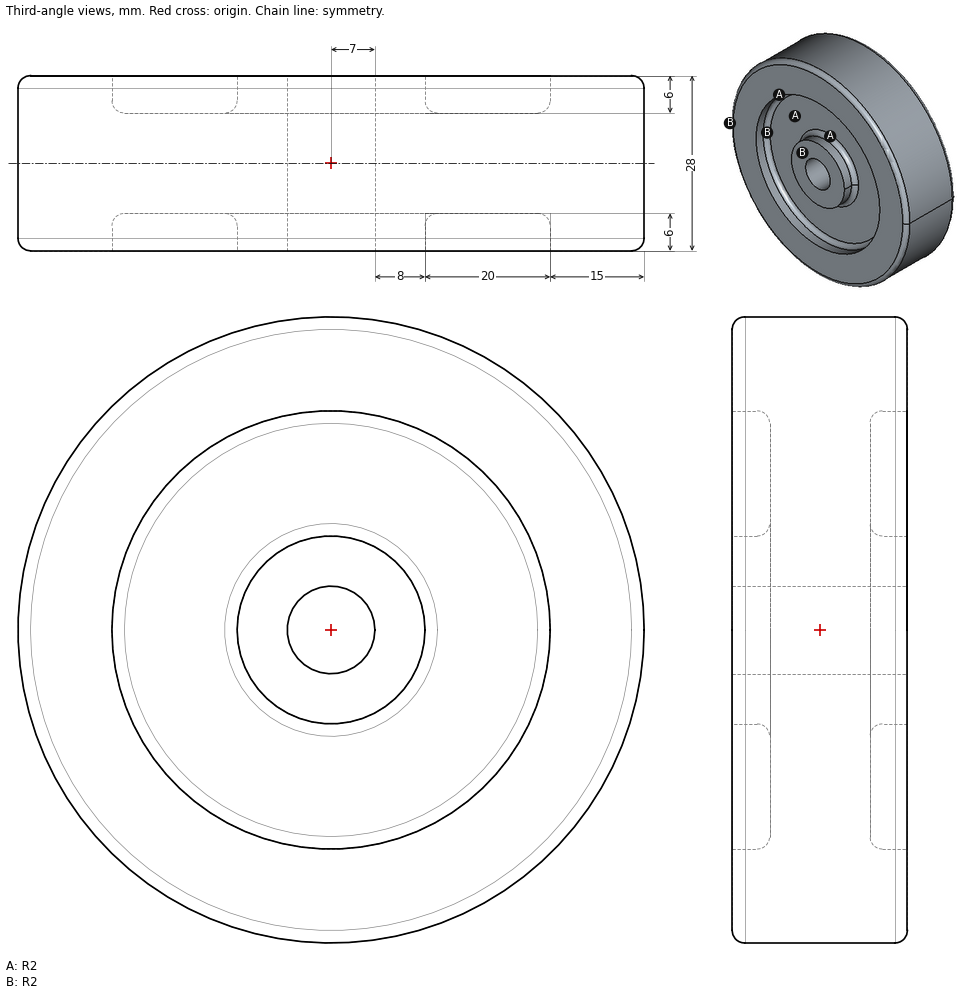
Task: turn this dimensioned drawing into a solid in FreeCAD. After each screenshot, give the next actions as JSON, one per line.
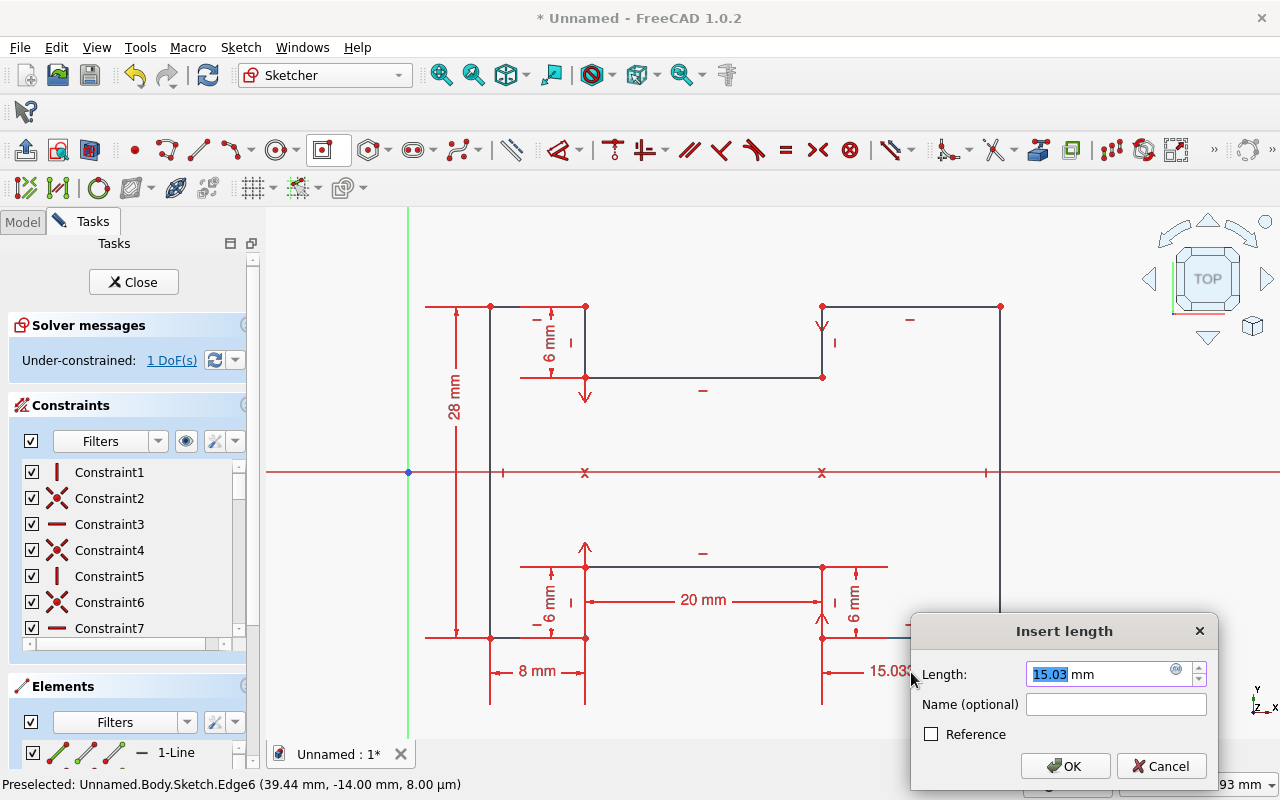
{"action": "type", "text": "15"}
{"action": "key", "text": "Return"}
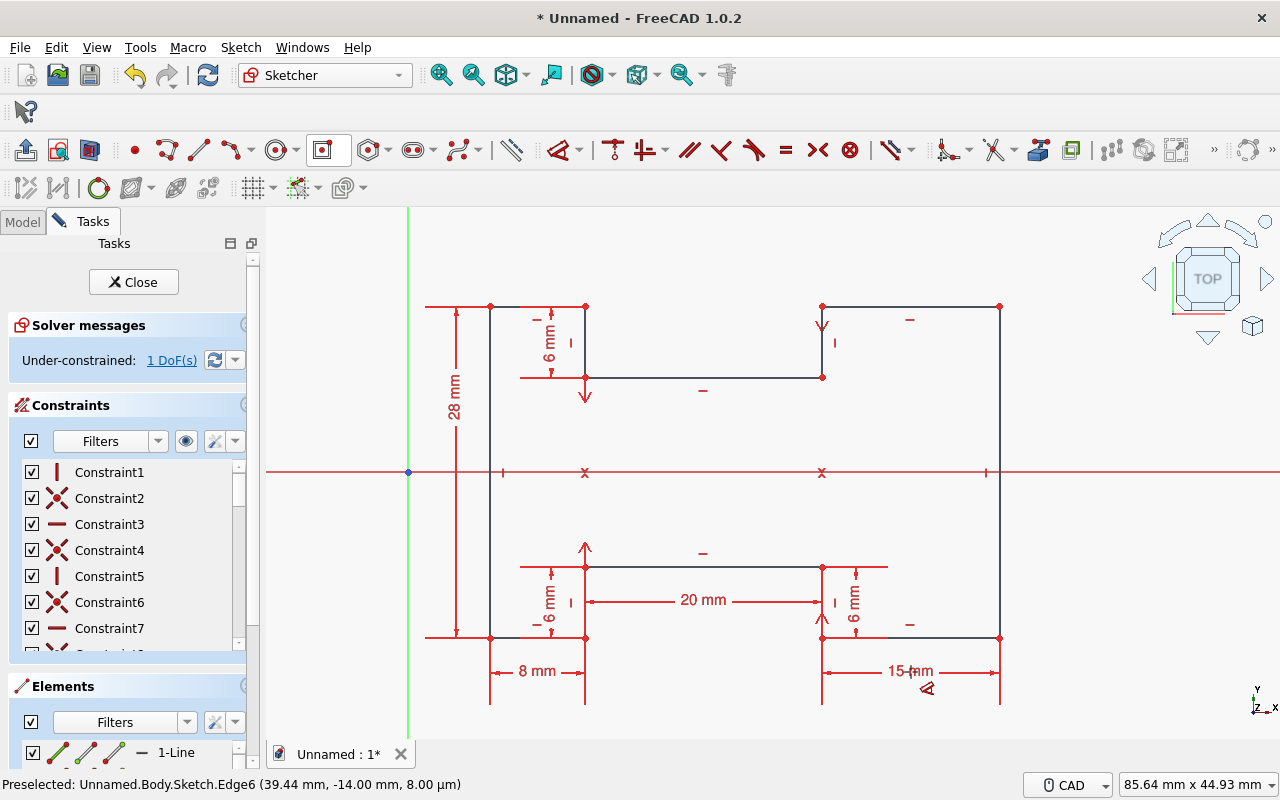
{"action": "left_click", "coordinate": [490, 307]}
{"action": "left_click", "coordinate": [449, 273]}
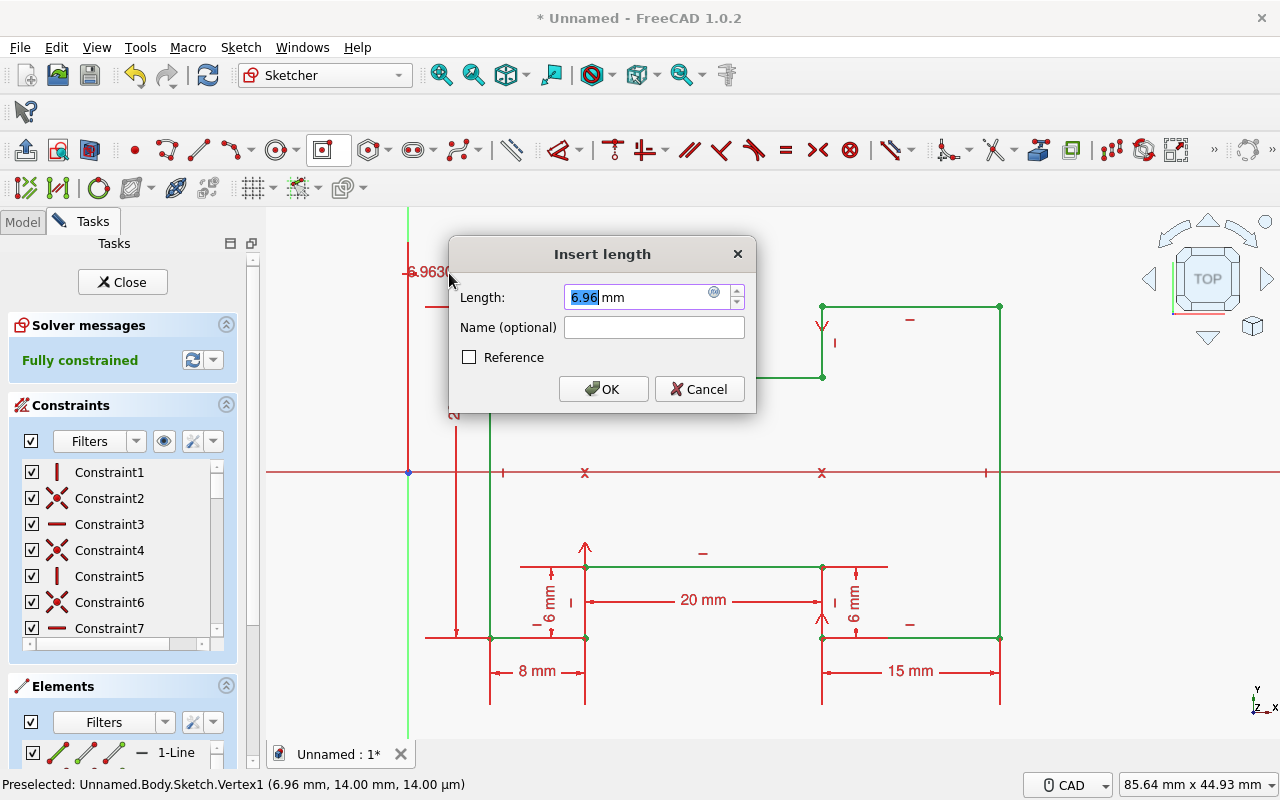
{"action": "type", "text": "7"}
{"action": "key", "text": "Return"}
{"action": "key", "text": "Escape"}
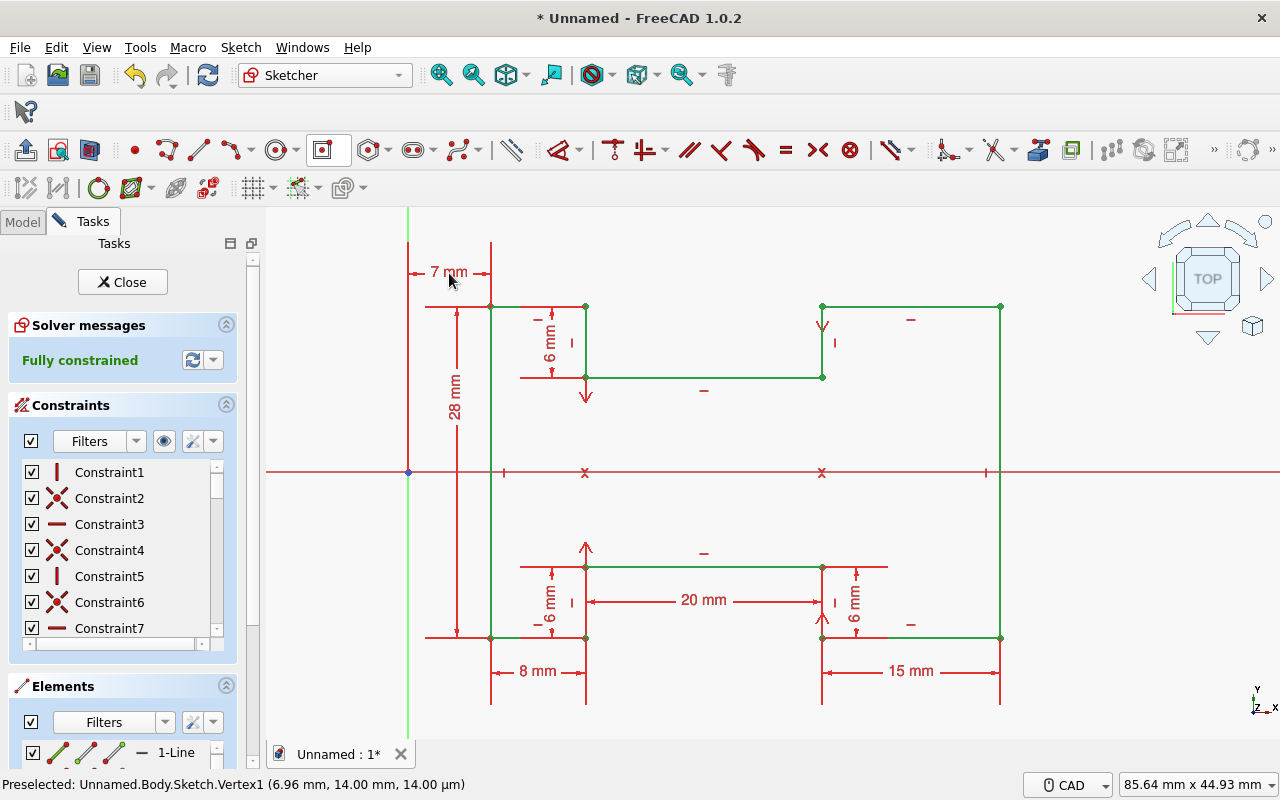
{"action": "left_click", "coordinate": [123, 282]}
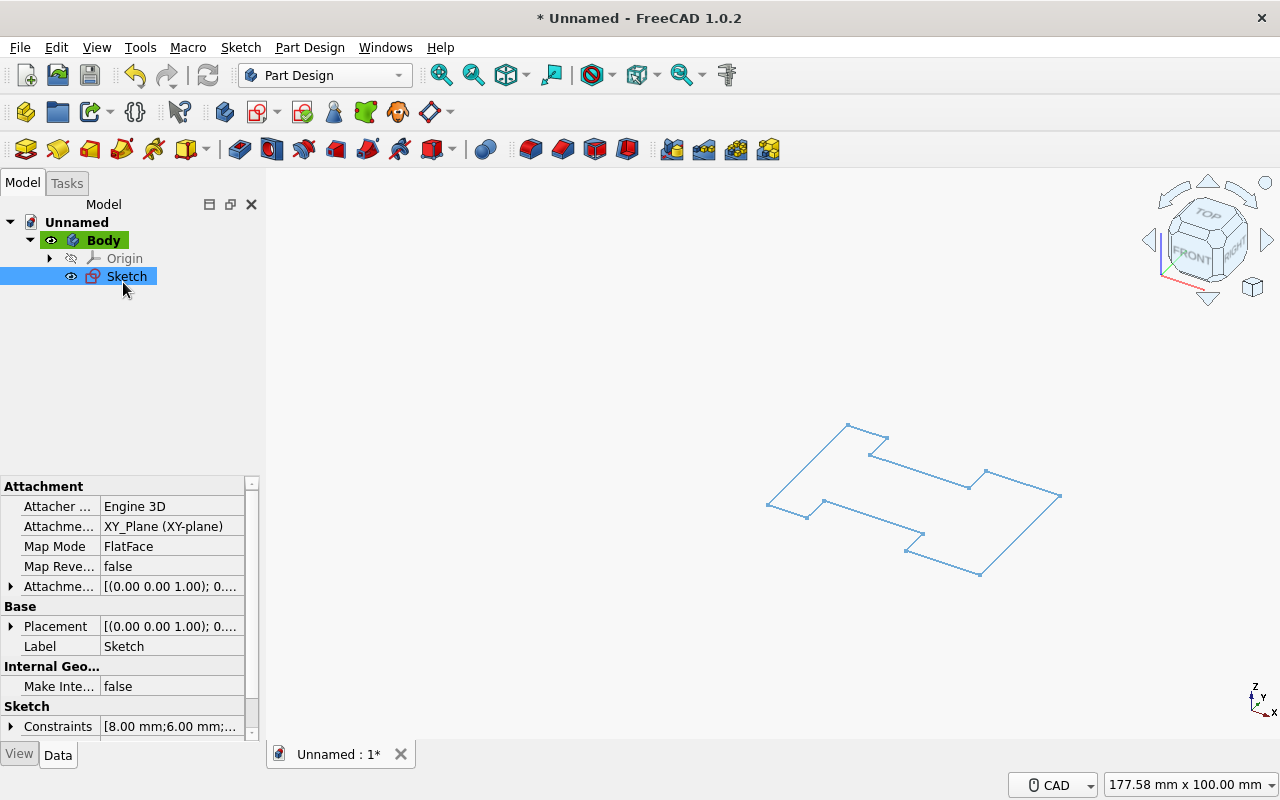
{"action": "left_click", "coordinate": [58, 150]}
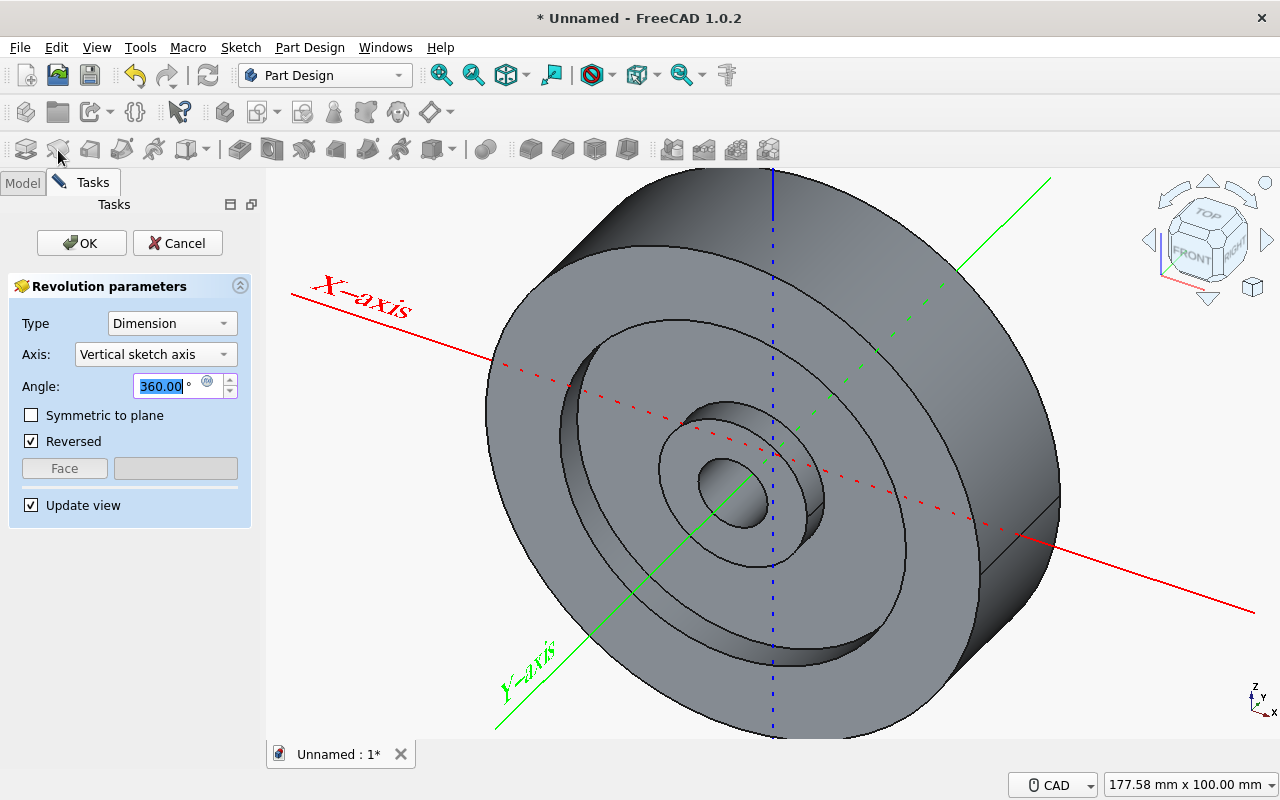
{"action": "left_click", "coordinate": [82, 243]}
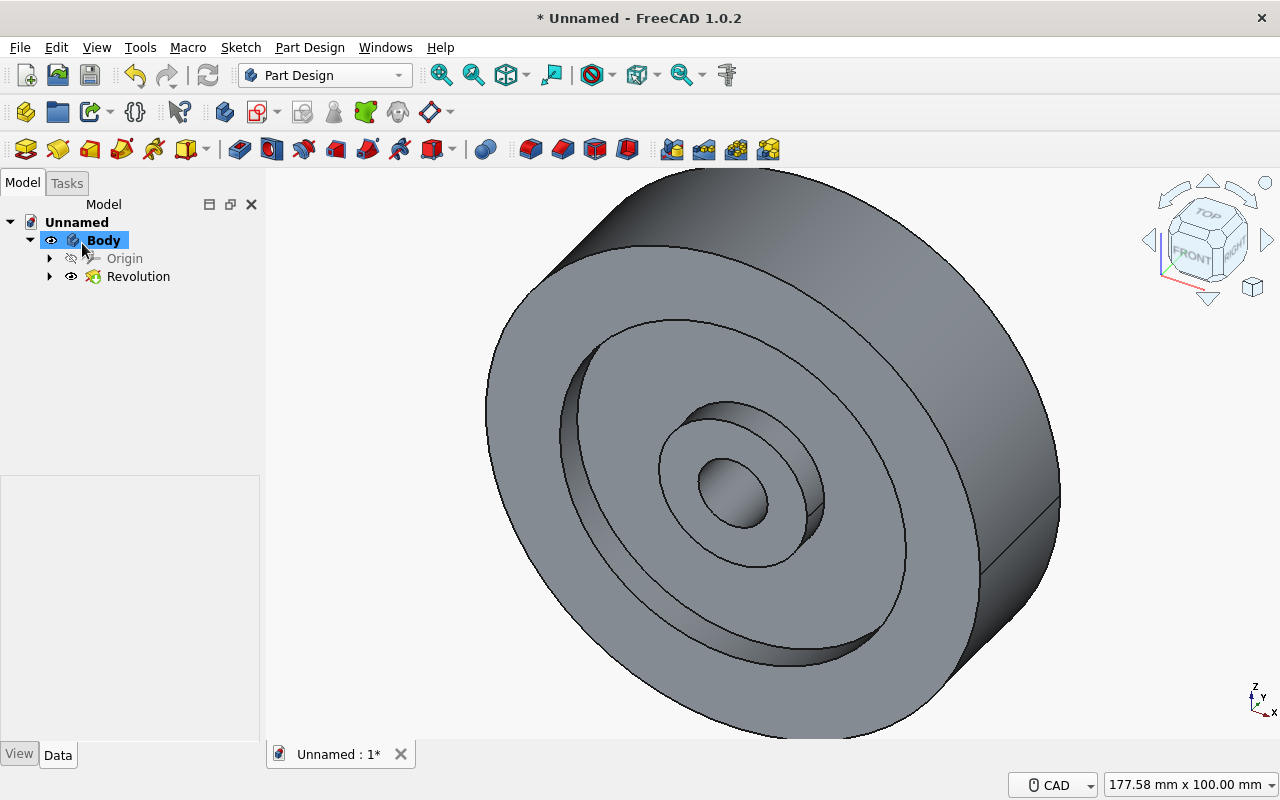
{"action": "left_click", "coordinate": [442, 76]}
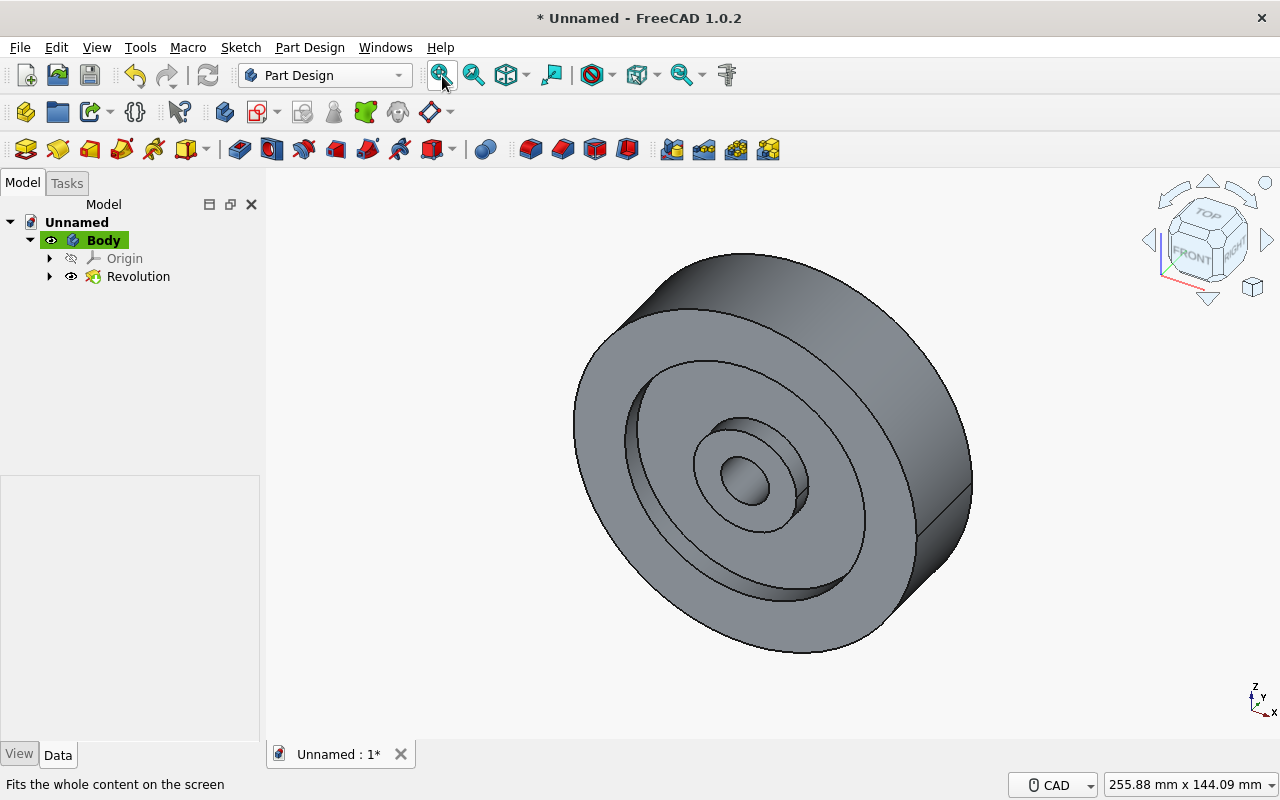
{"action": "key", "text": "0"}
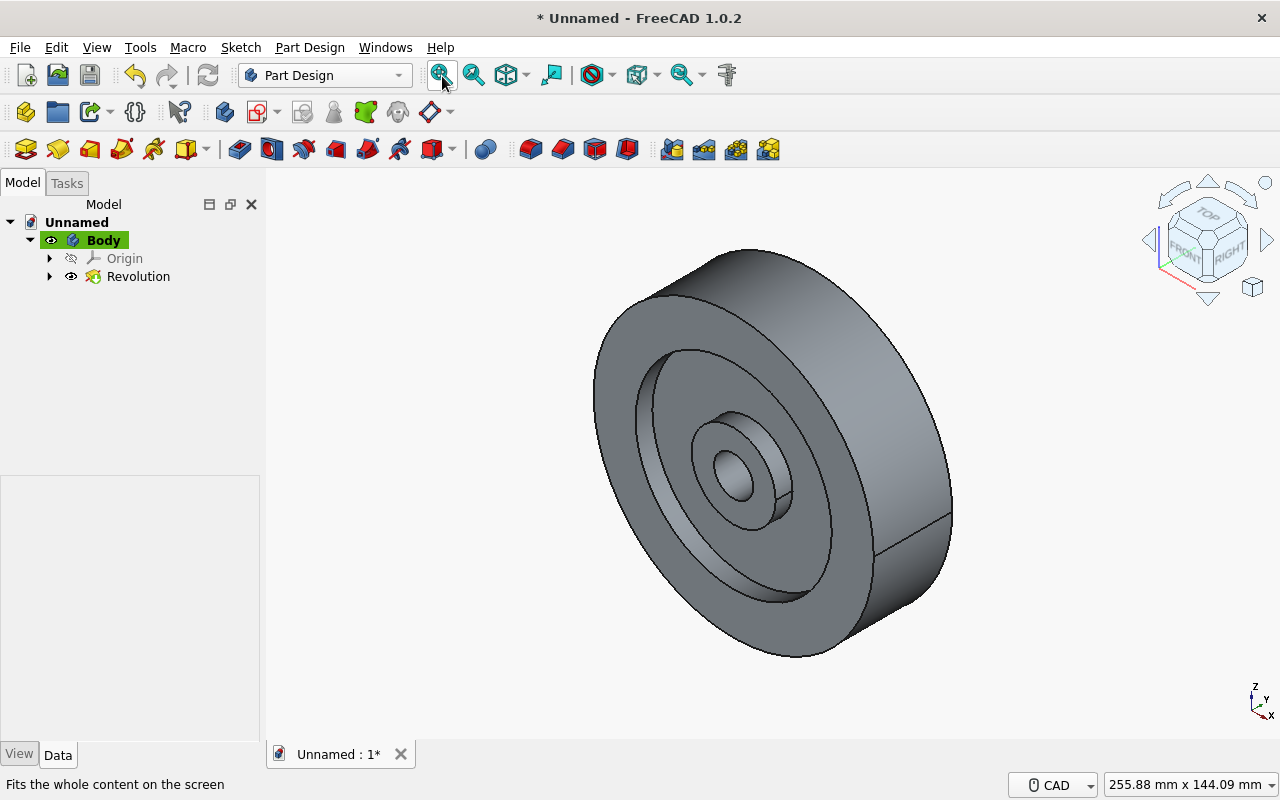
{"action": "key", "text": "2"}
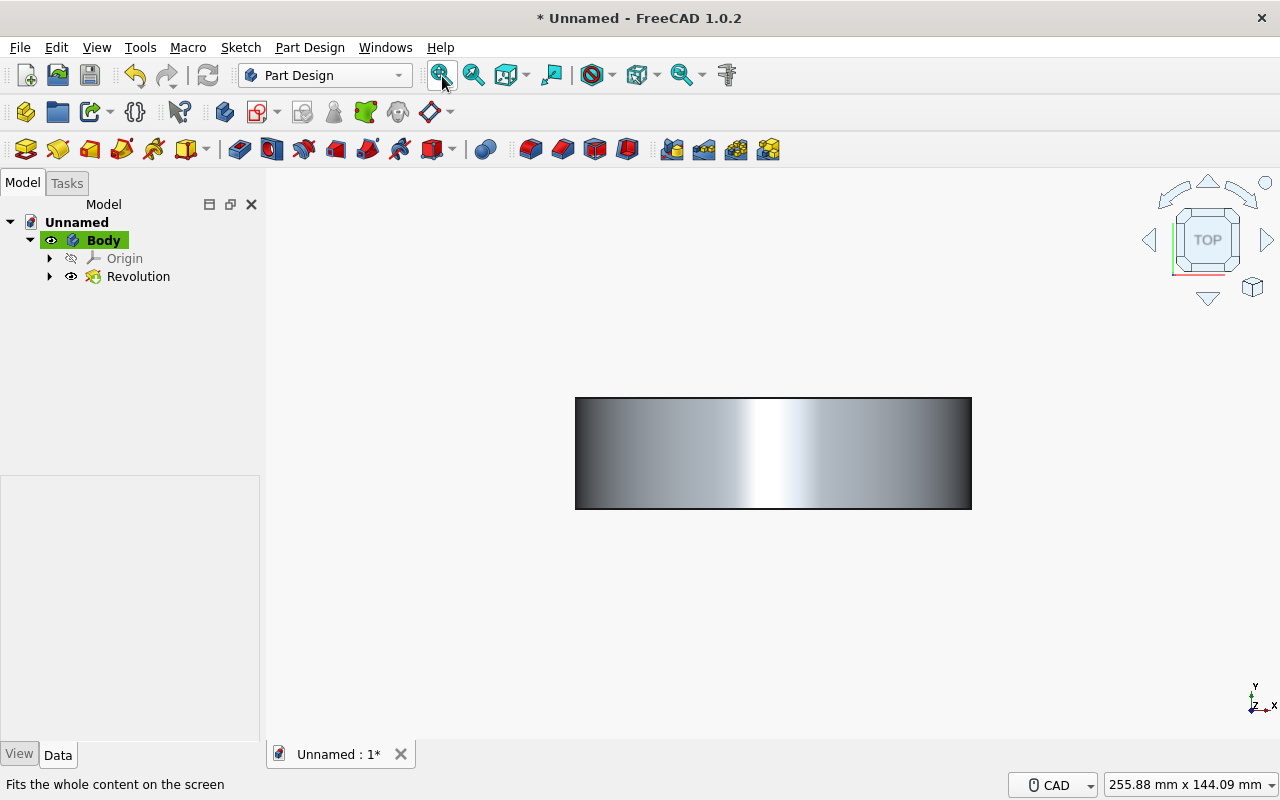
{"action": "left_click", "coordinate": [442, 76]}